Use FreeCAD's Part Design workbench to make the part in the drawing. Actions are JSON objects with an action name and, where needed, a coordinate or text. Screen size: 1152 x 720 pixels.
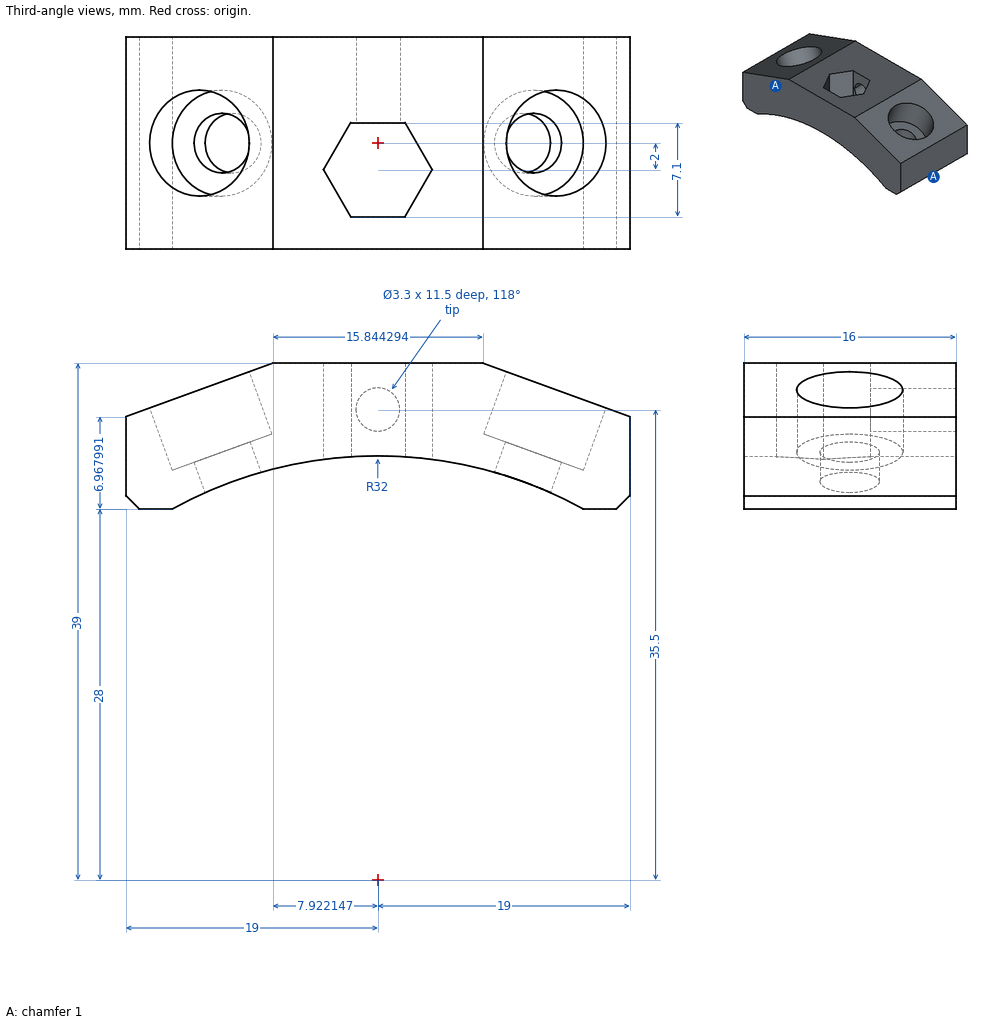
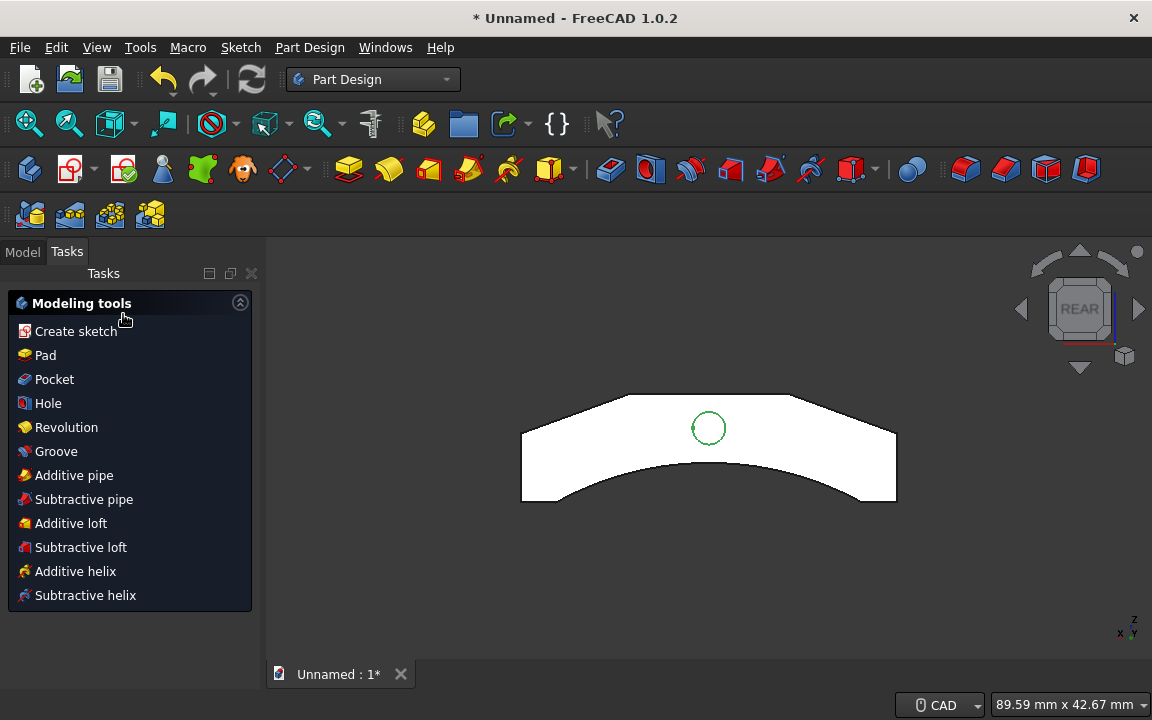
{"action": "left_click", "coordinate": [652, 170]}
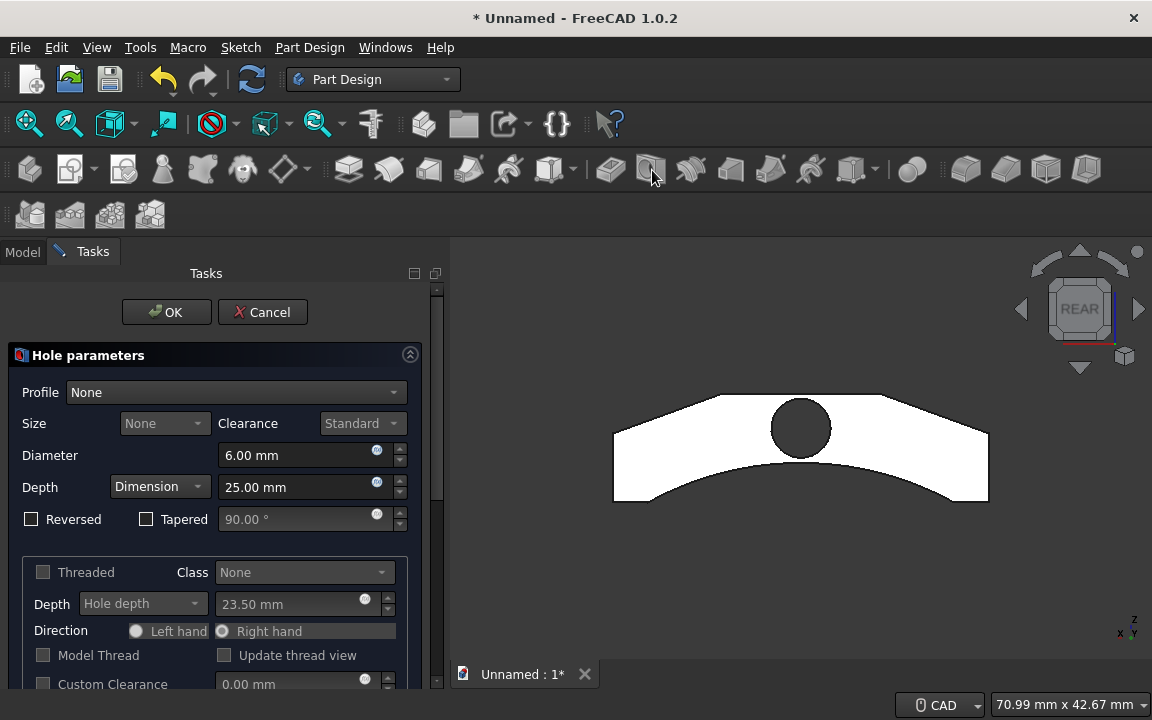
{"action": "triple_click", "coordinate": [305, 455]}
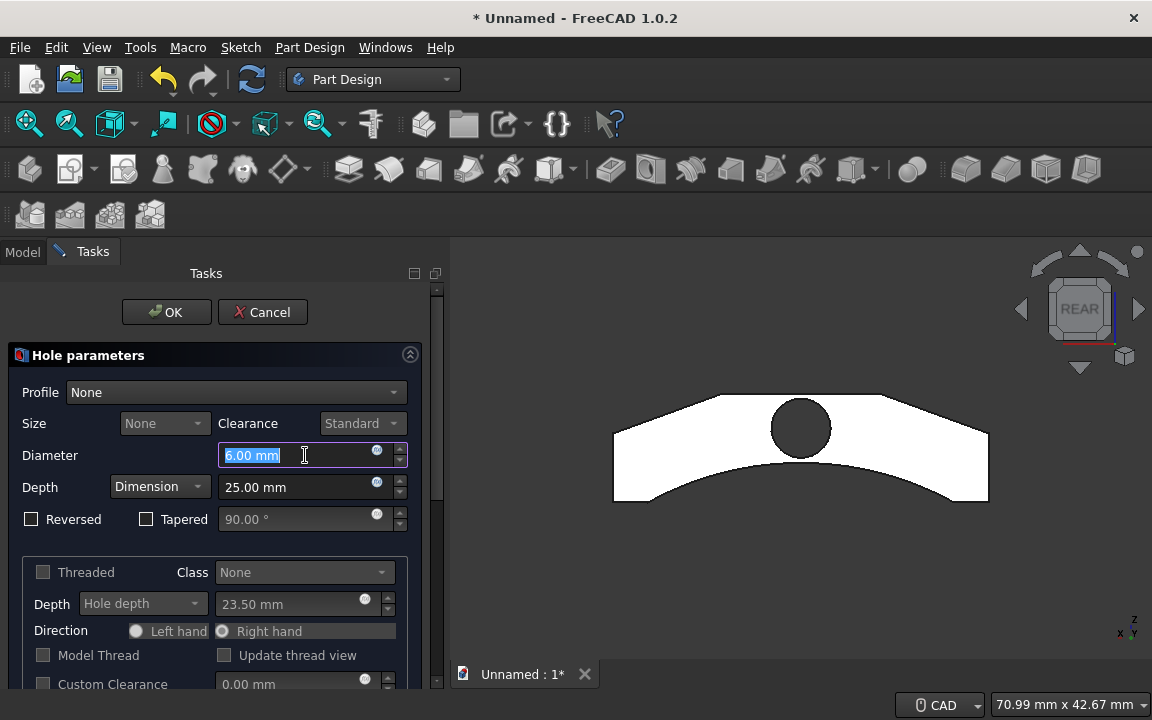
{"action": "type", "text": "3.3"}
{"action": "key", "text": "Tab"}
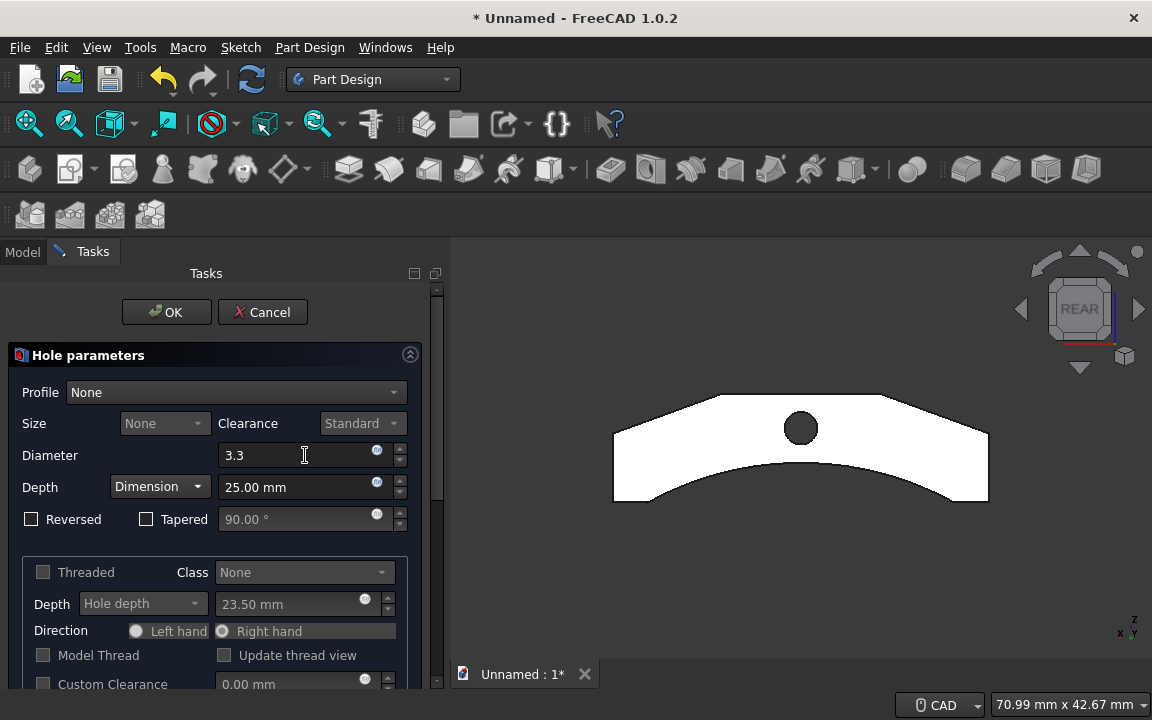
{"action": "triple_click", "coordinate": [305, 487]}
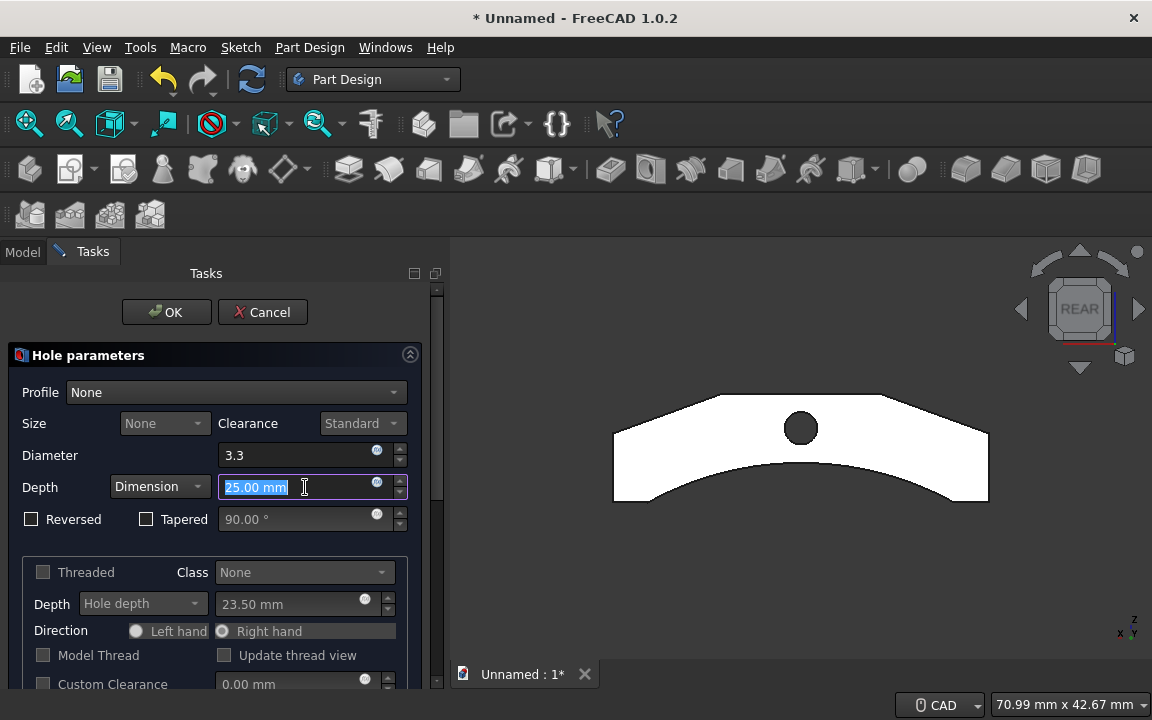
{"action": "type", "text": "11.5"}
{"action": "key", "text": "Tab"}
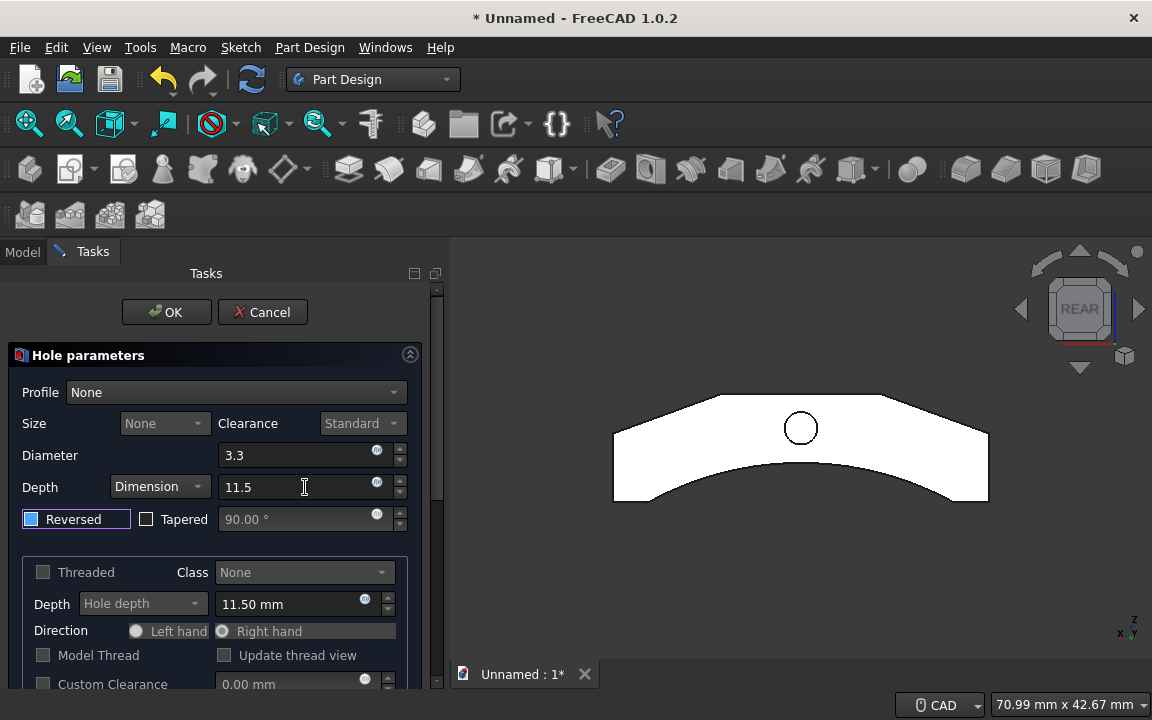
{"action": "left_click", "coordinate": [167, 312]}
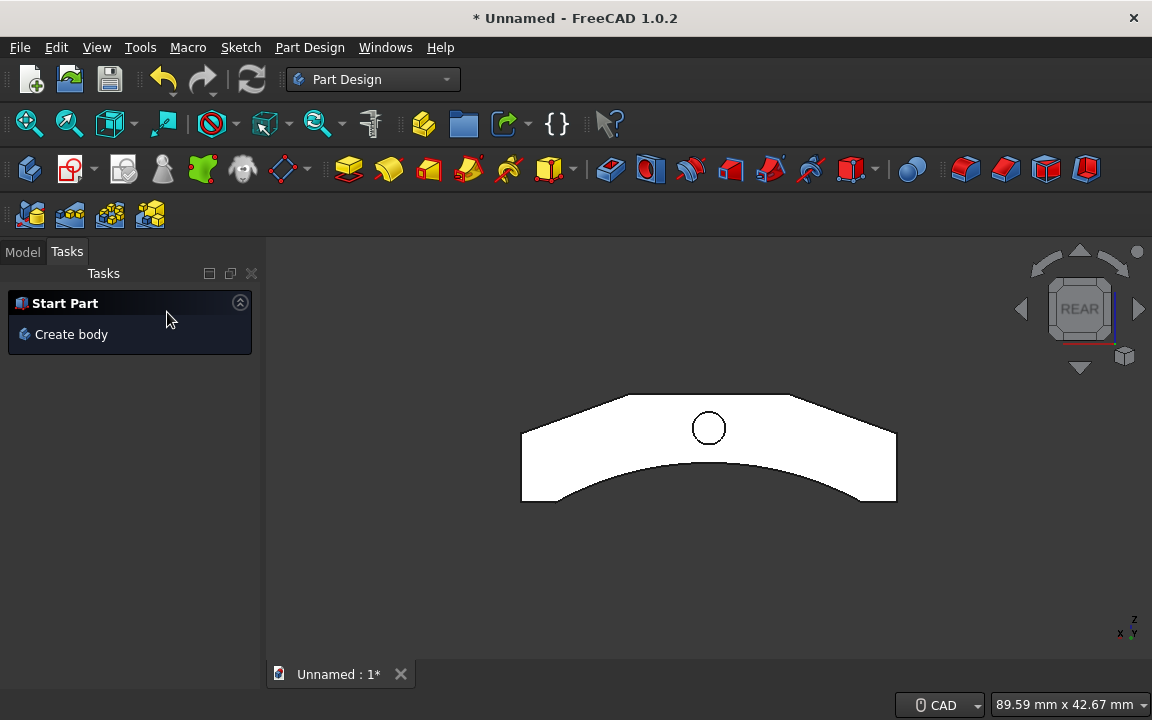
{"action": "left_click", "coordinate": [30, 124]}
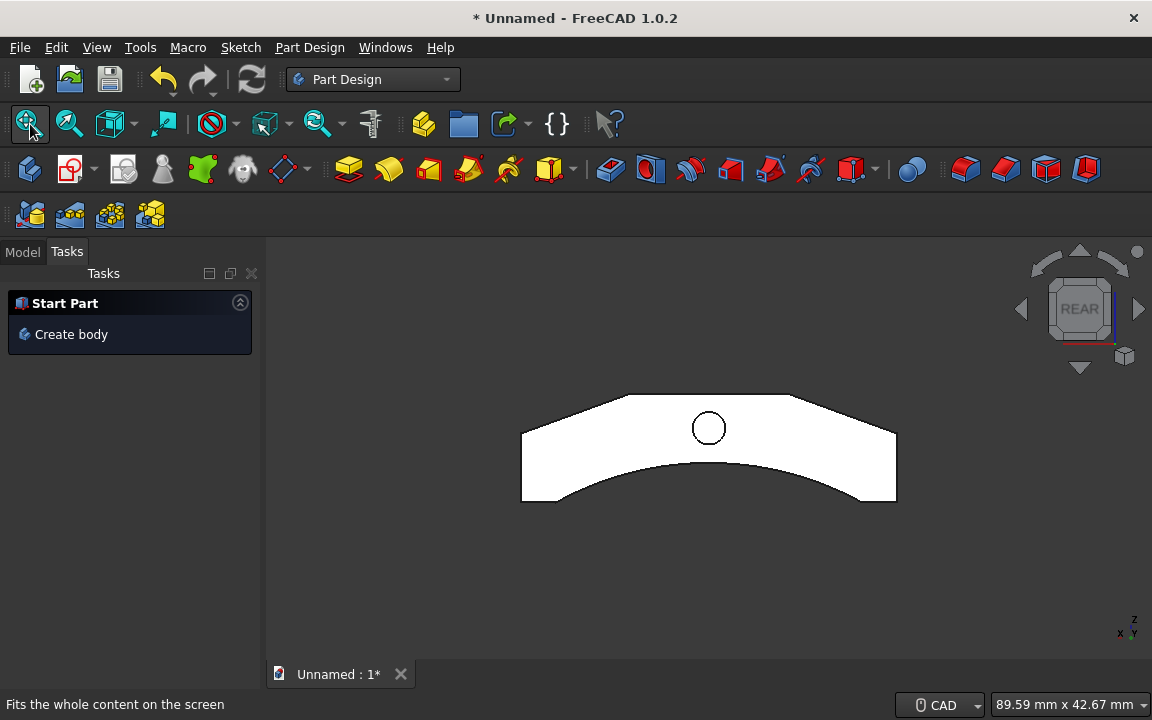
{"action": "key", "text": "0"}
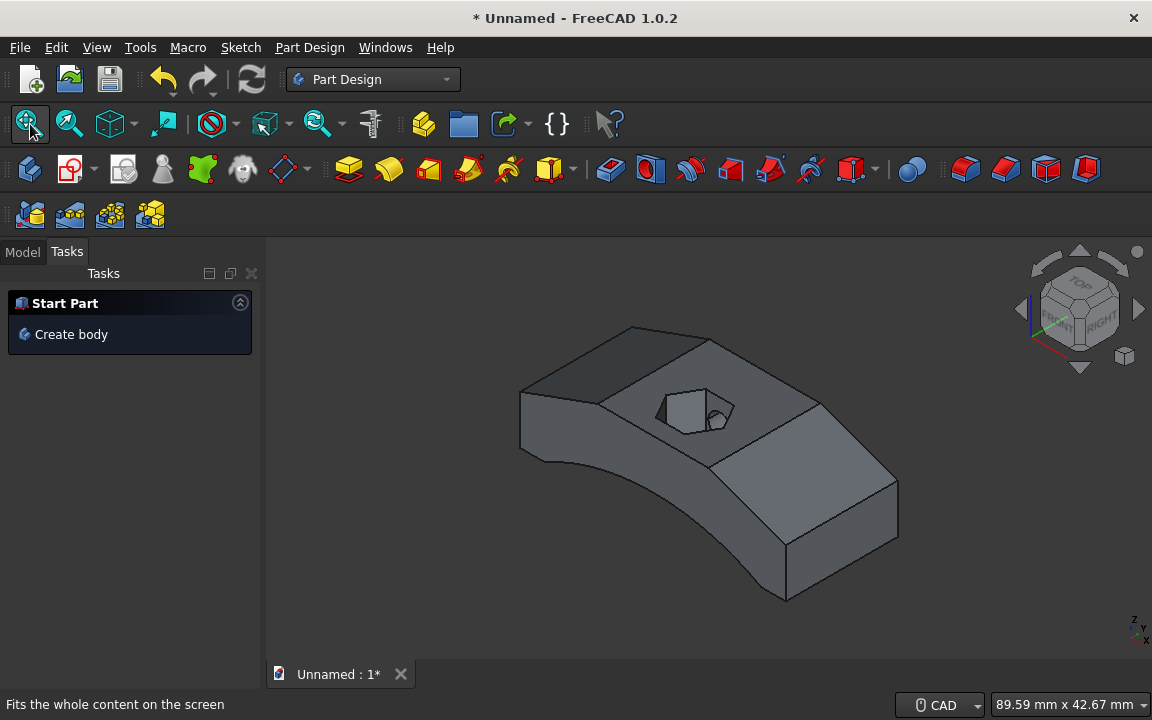
{"action": "left_click", "coordinate": [615, 365]}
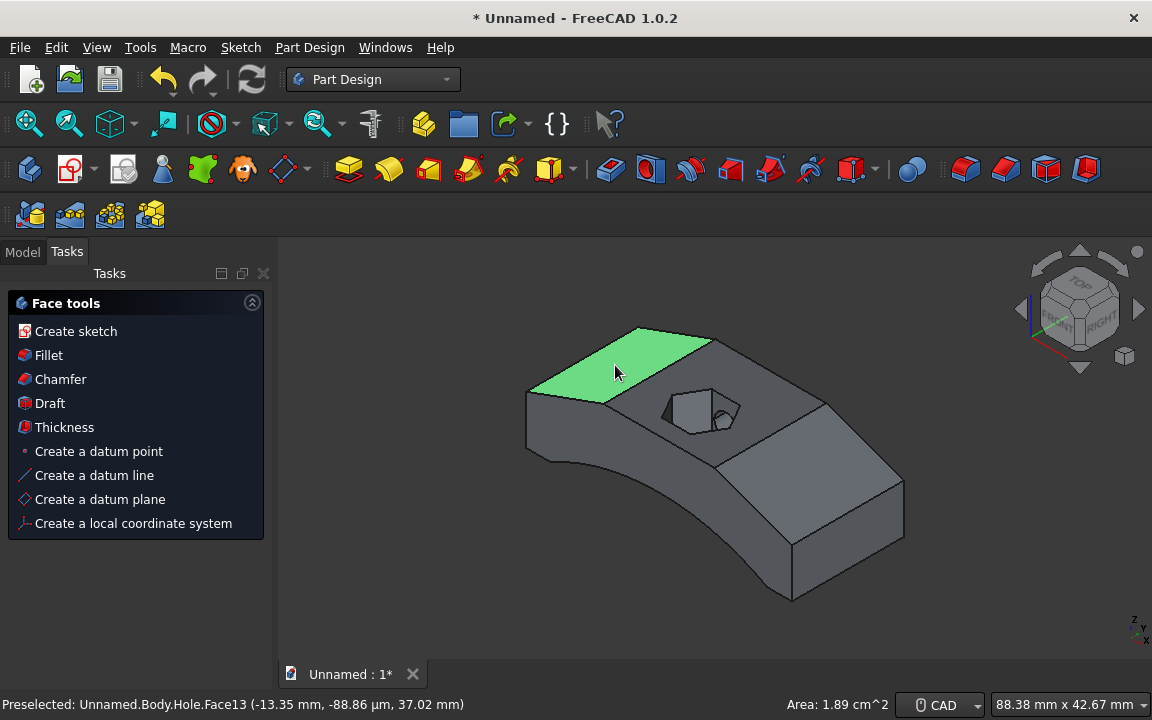
{"action": "left_click", "coordinate": [70, 170]}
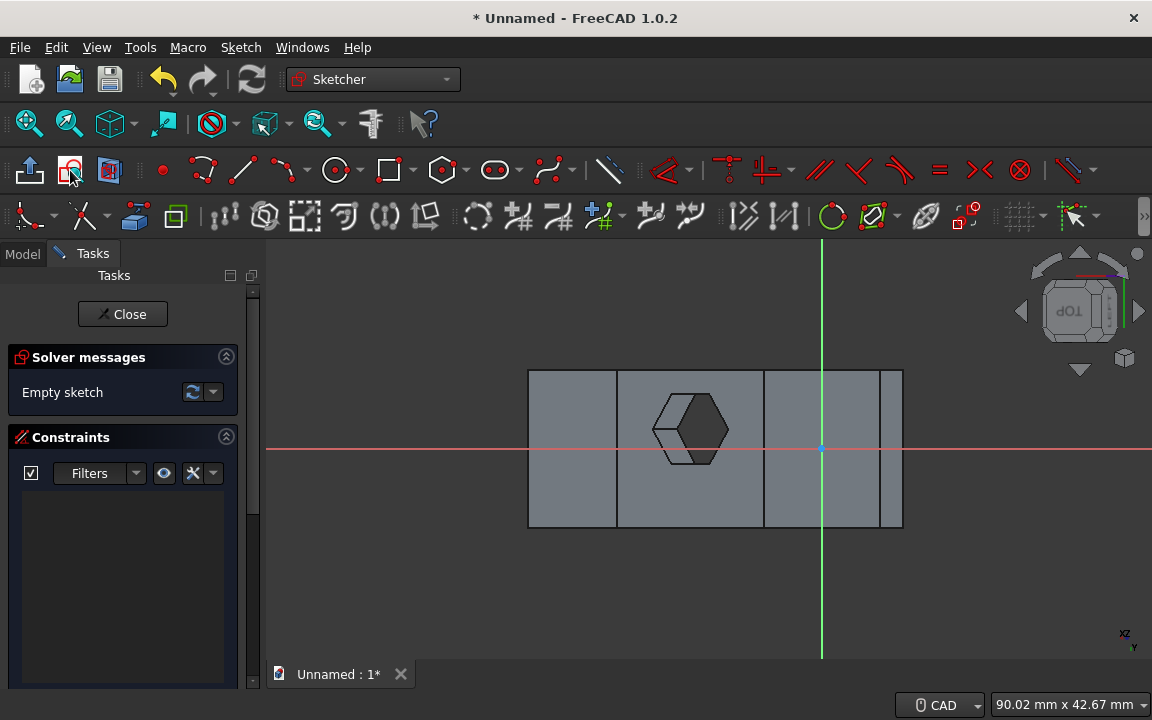
{"action": "key", "text": "q s"}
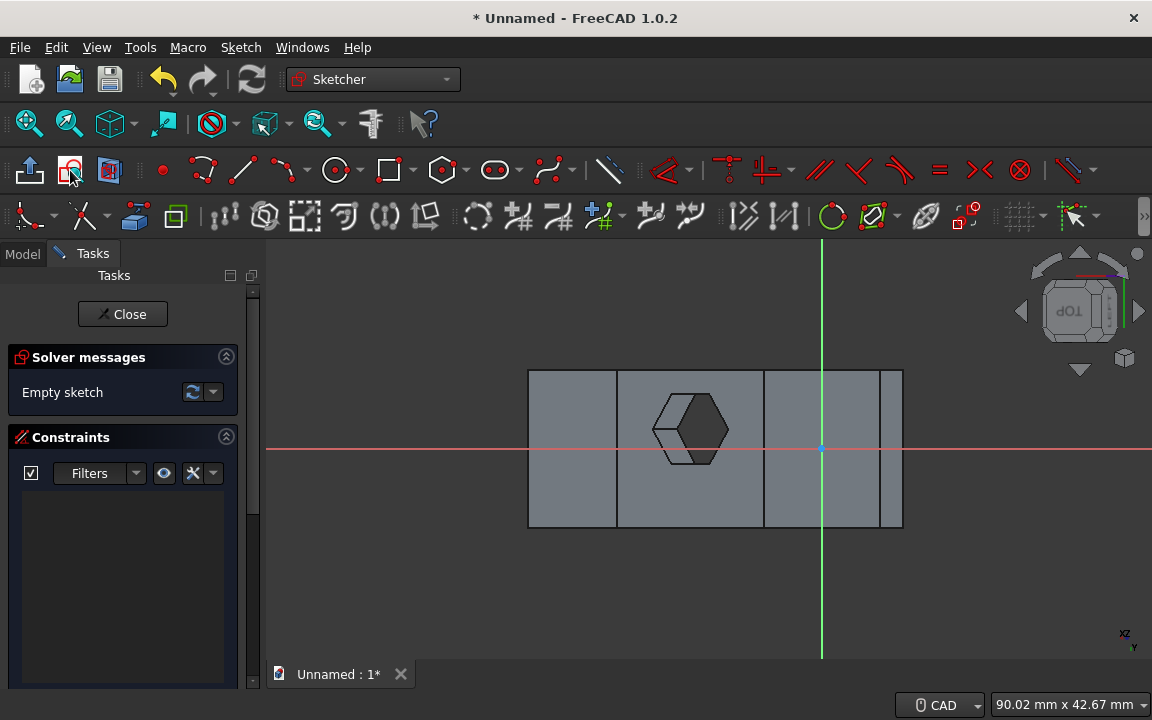
{"action": "scroll", "coordinate": [858, 449], "scroll_direction": "up", "scroll_amount": 9}